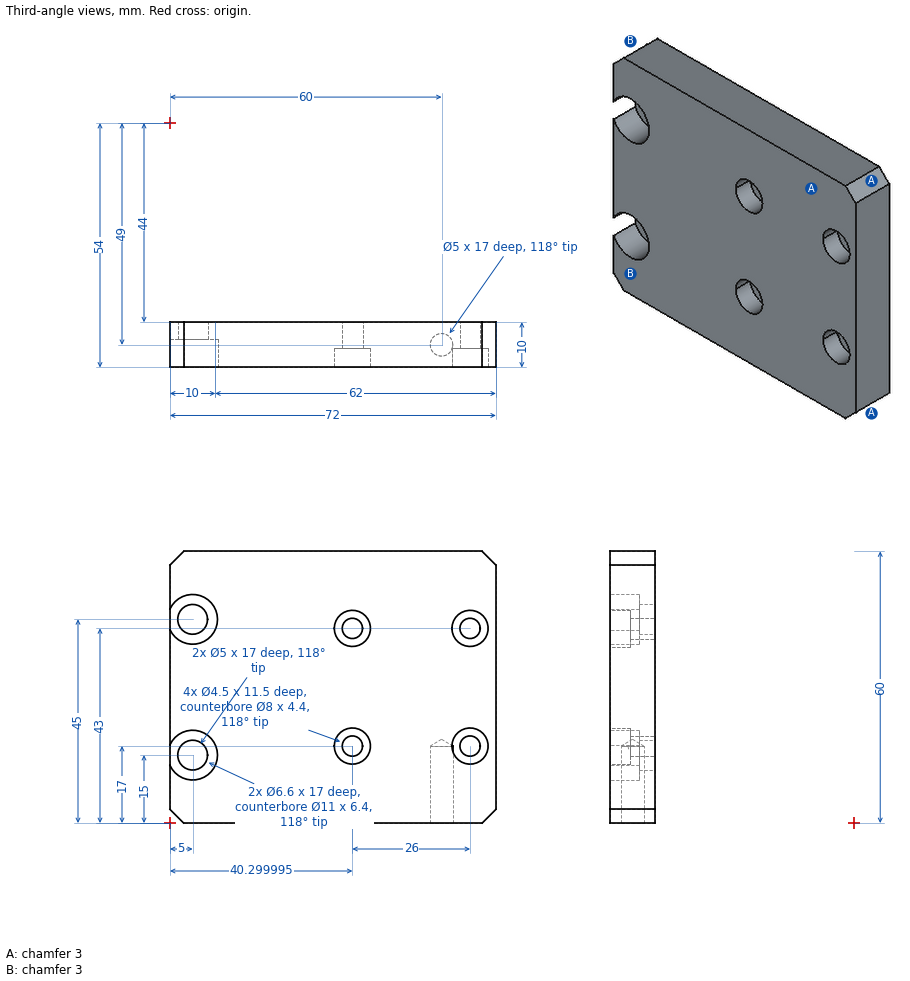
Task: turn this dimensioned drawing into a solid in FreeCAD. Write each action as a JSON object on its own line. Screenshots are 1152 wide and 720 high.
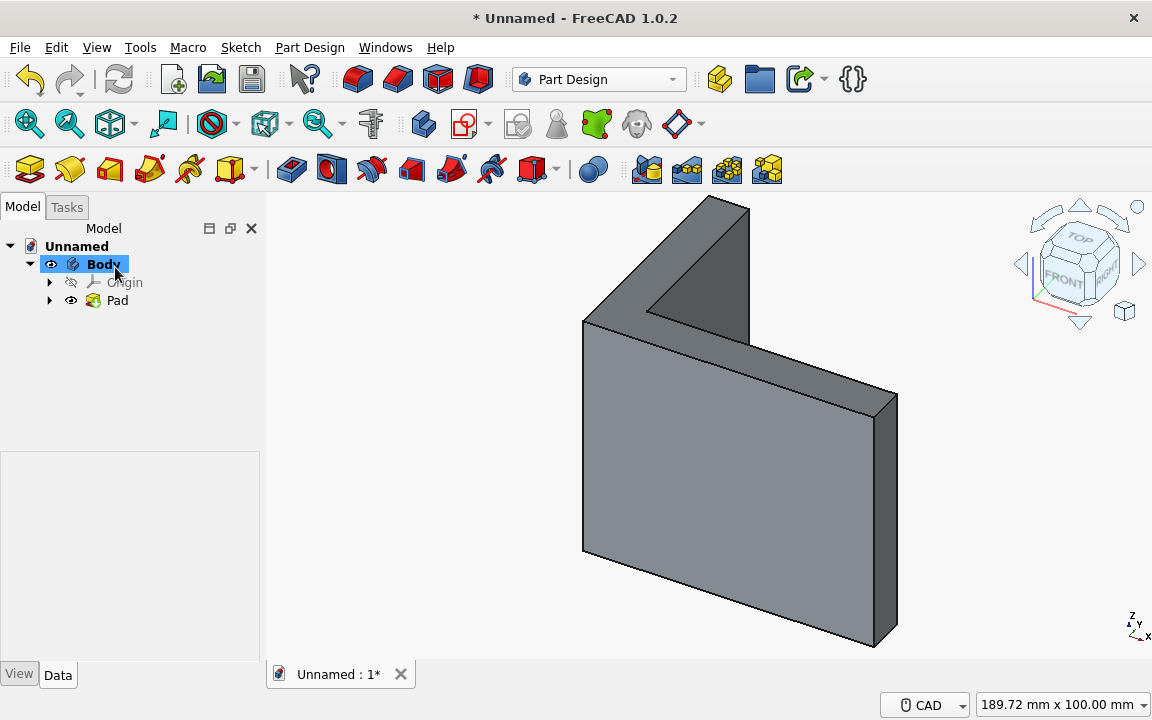
{"action": "key", "text": "5"}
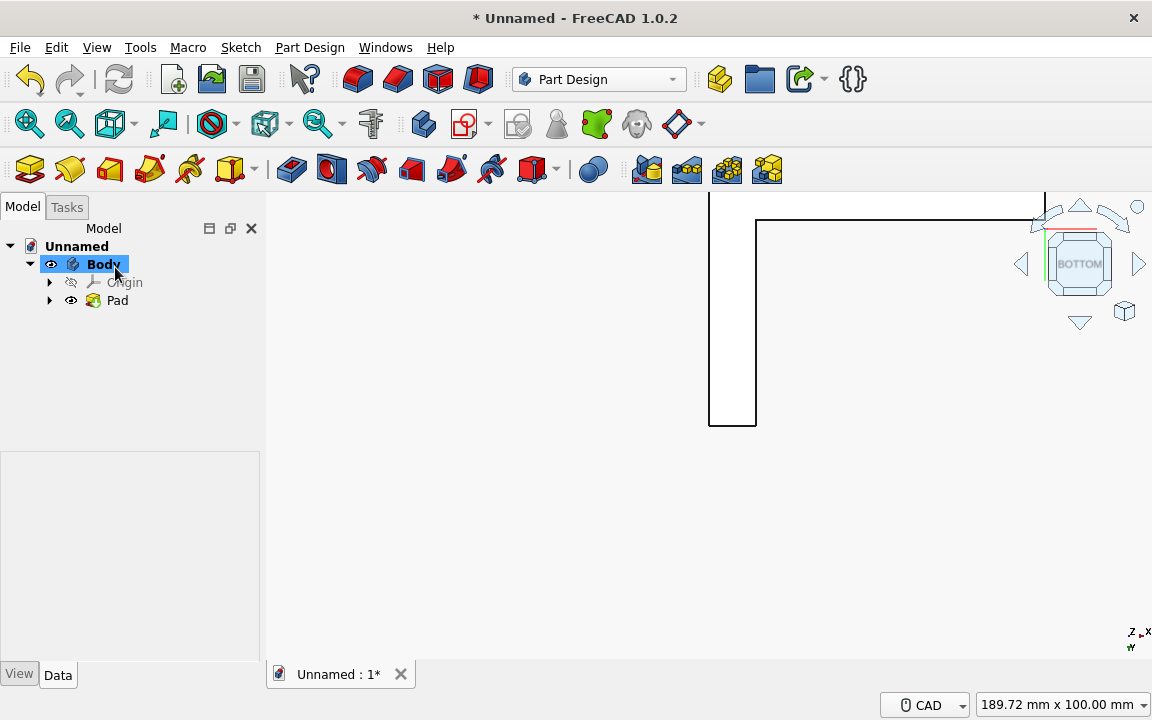
{"action": "left_click", "coordinate": [30, 124]}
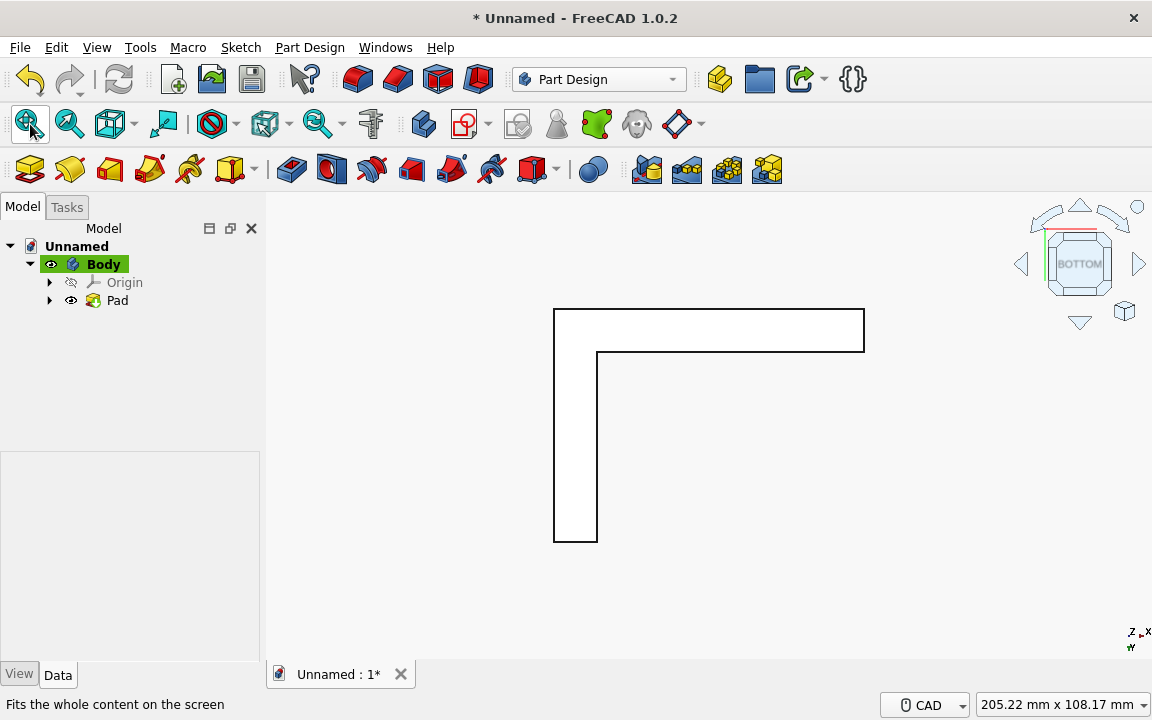
{"action": "left_click", "coordinate": [576, 491]}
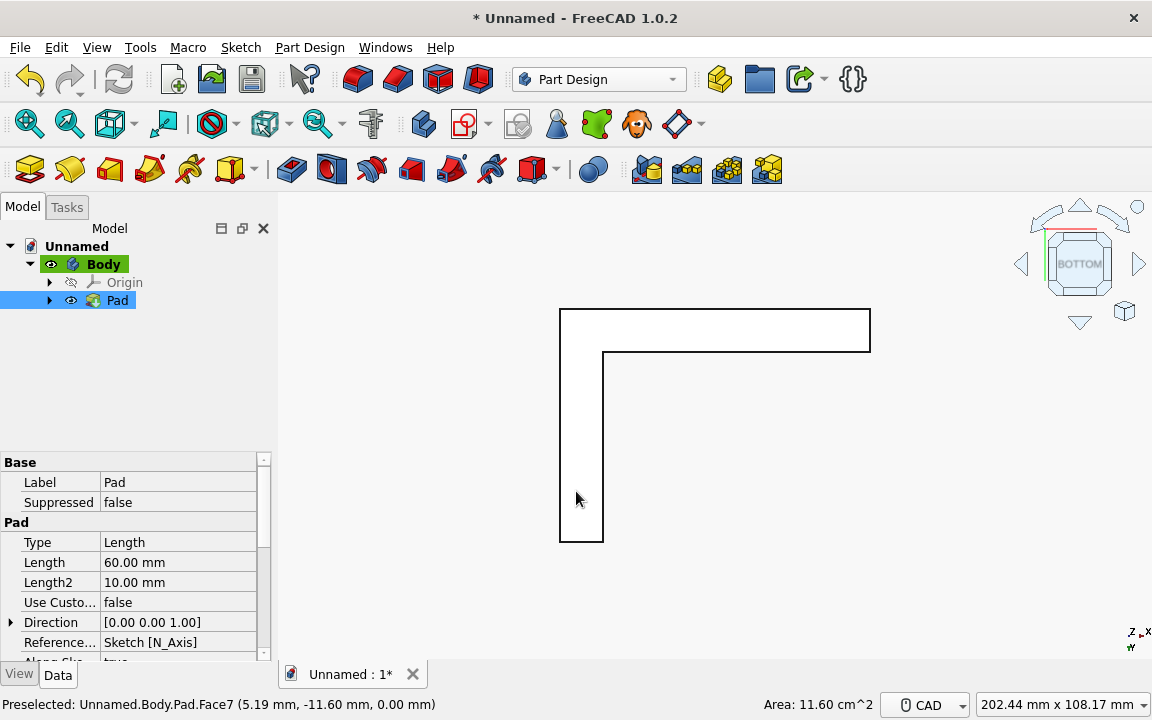
{"action": "left_click", "coordinate": [464, 124]}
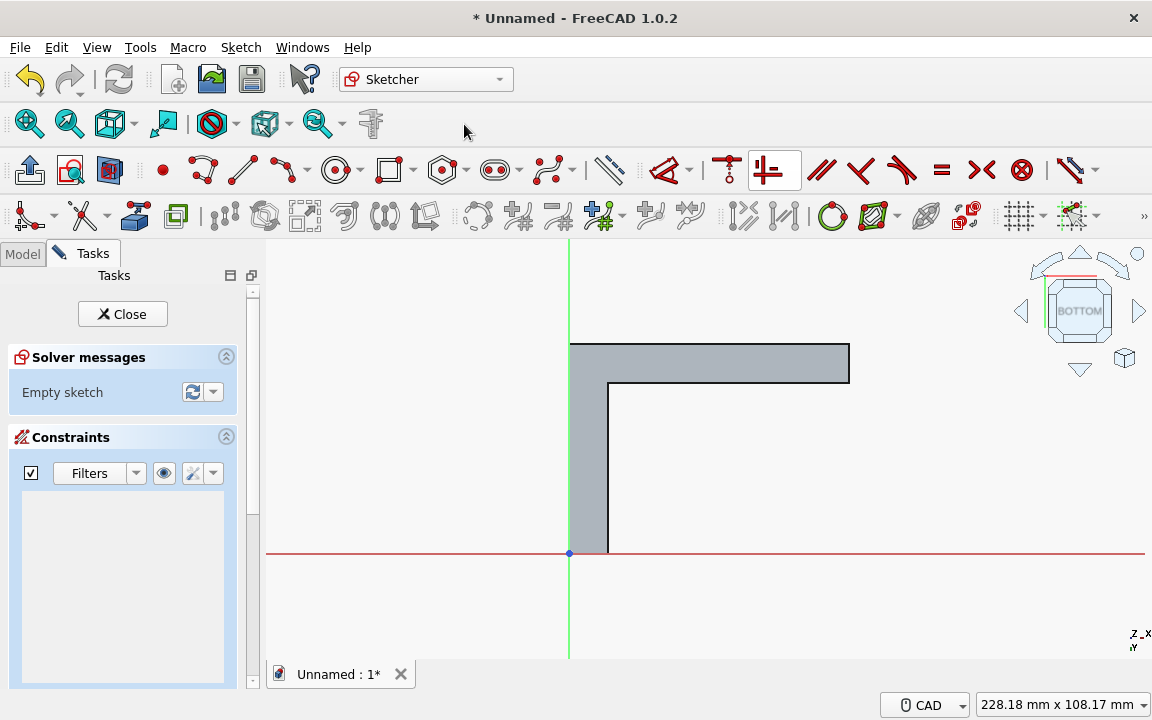
{"action": "scroll", "coordinate": [815, 357], "scroll_direction": "up", "scroll_amount": 13}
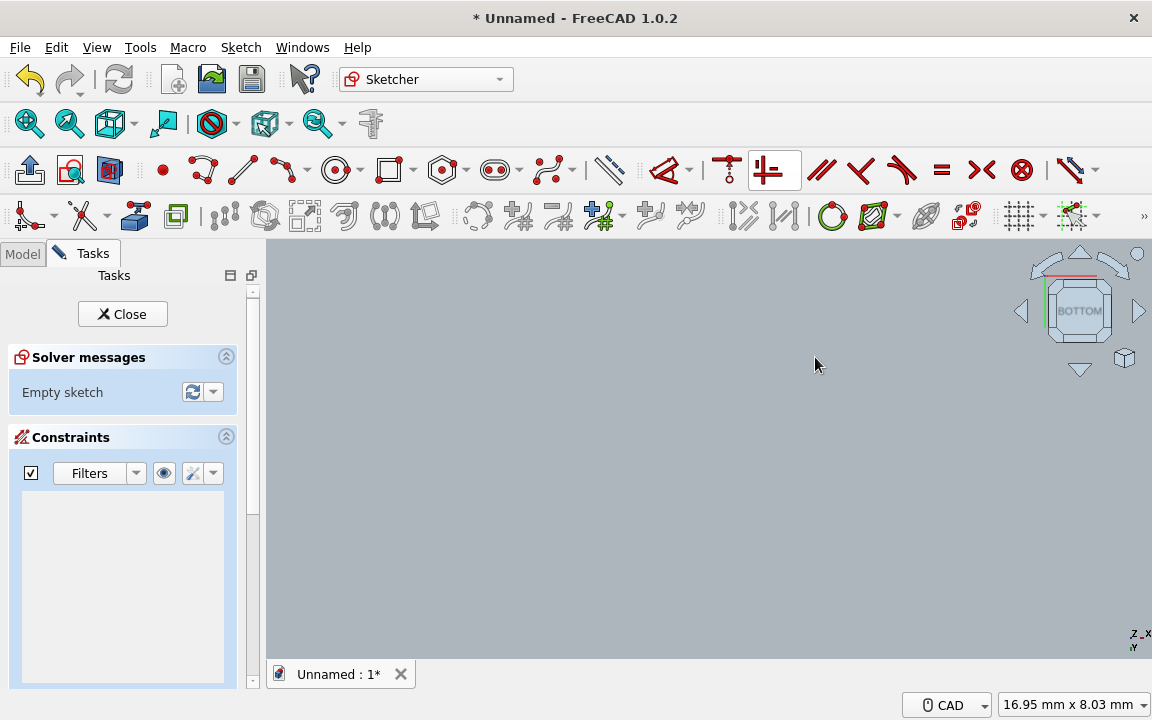
{"action": "left_click", "coordinate": [336, 170]}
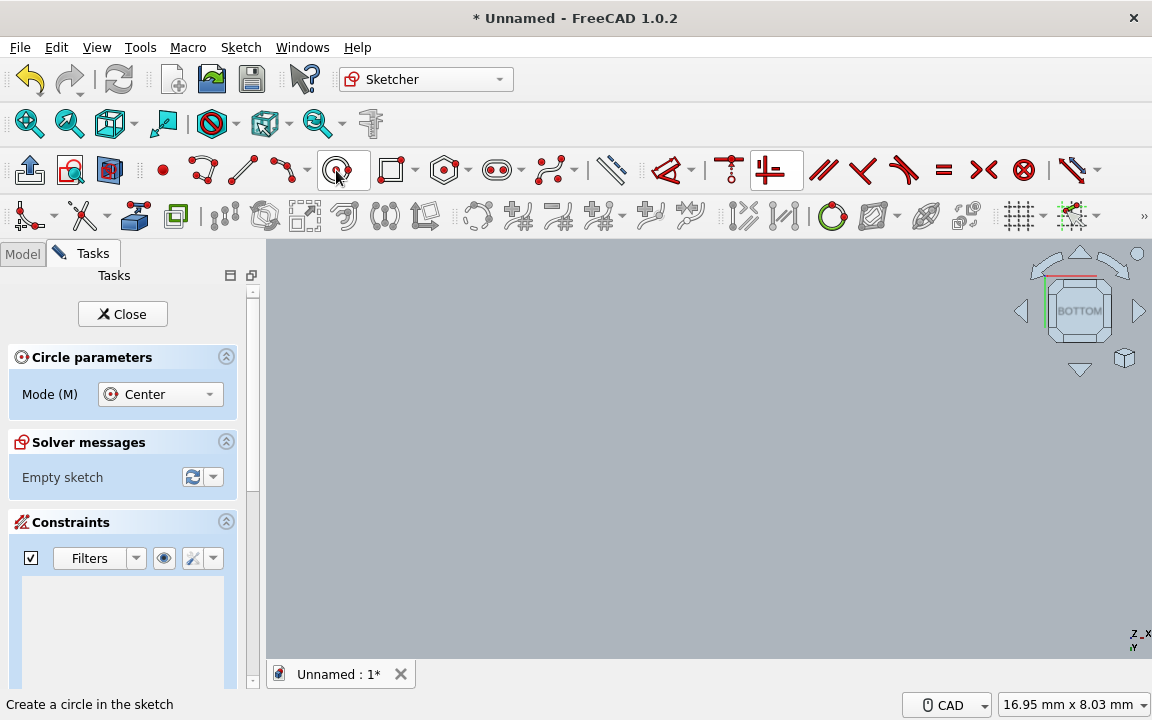
{"action": "left_click", "coordinate": [635, 442]}
{"action": "left_click", "coordinate": [727, 350]}
{"action": "key", "text": "Escape"}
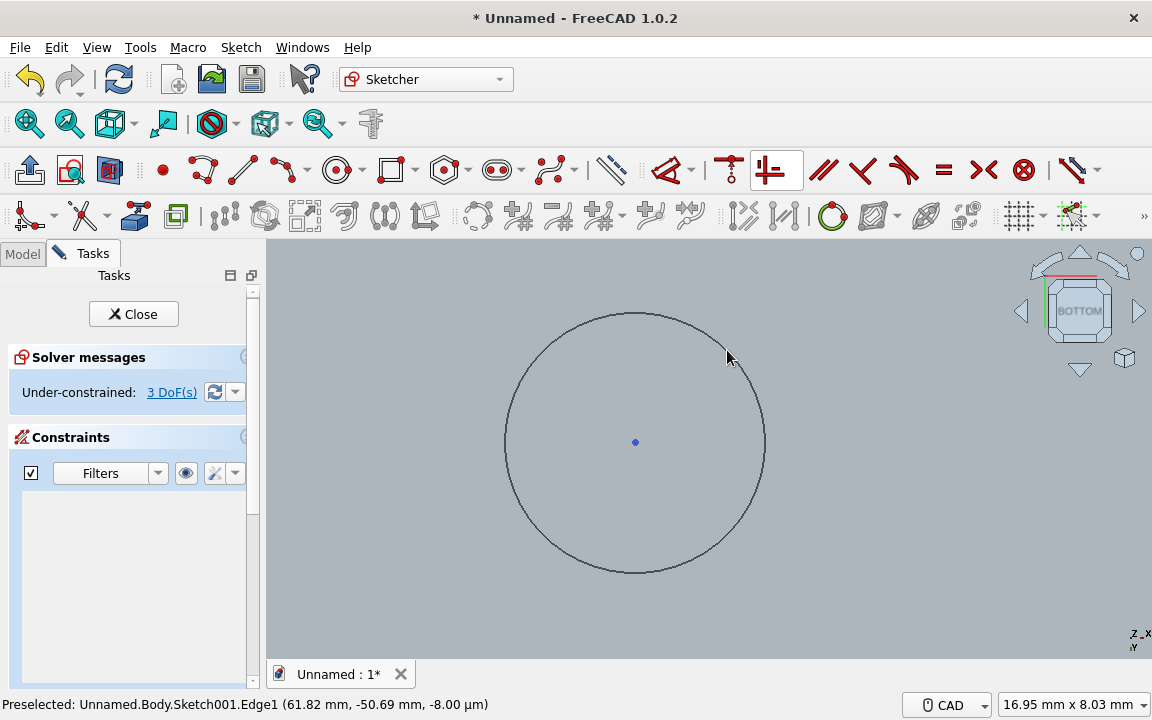
{"action": "left_click", "coordinate": [666, 170]}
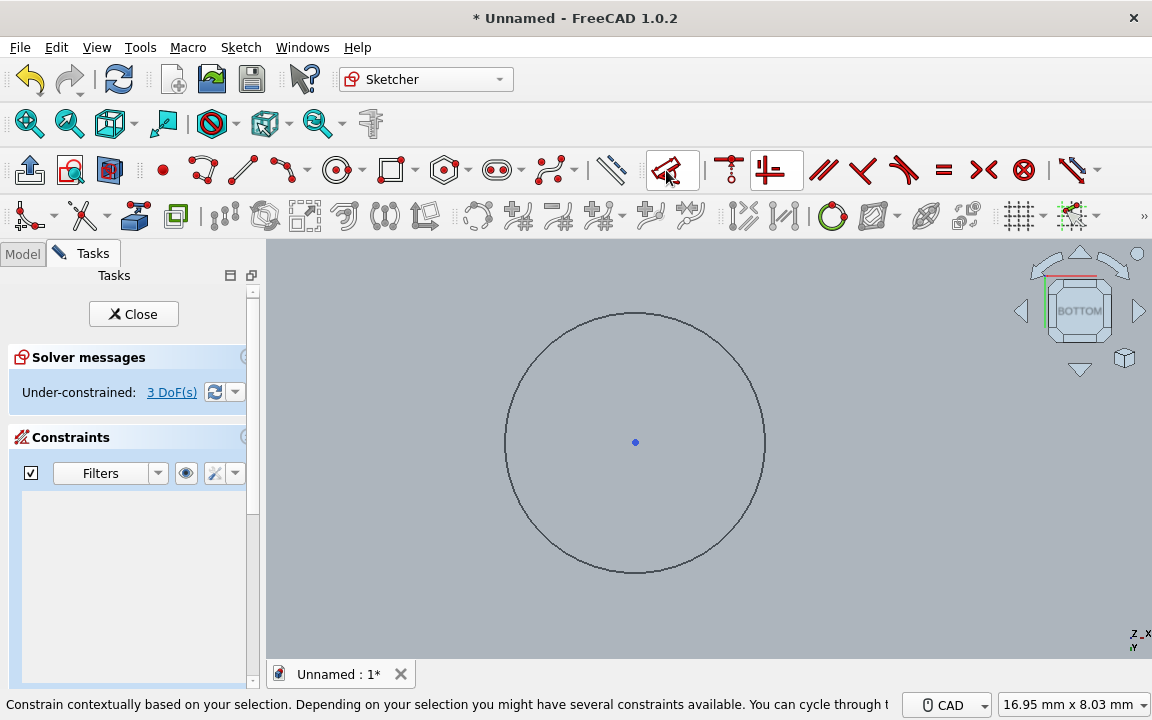
{"action": "left_click", "coordinate": [727, 351]}
{"action": "left_click", "coordinate": [750, 328]}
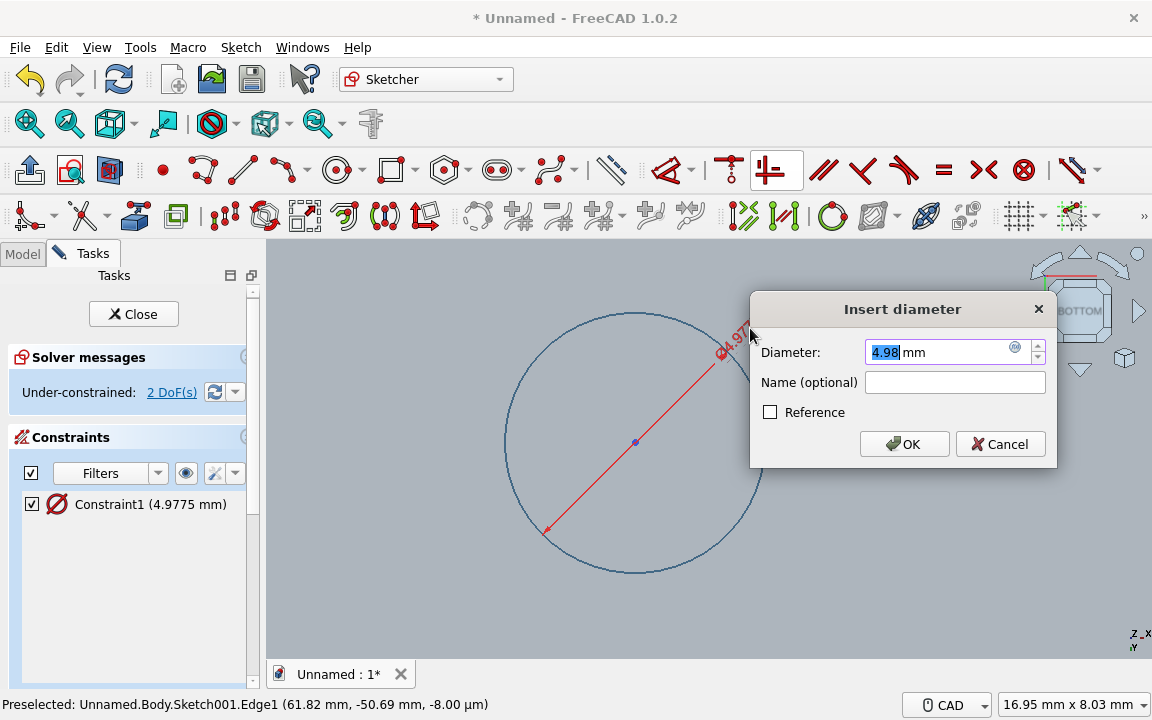
{"action": "type", "text": "5"}
{"action": "key", "text": "Return"}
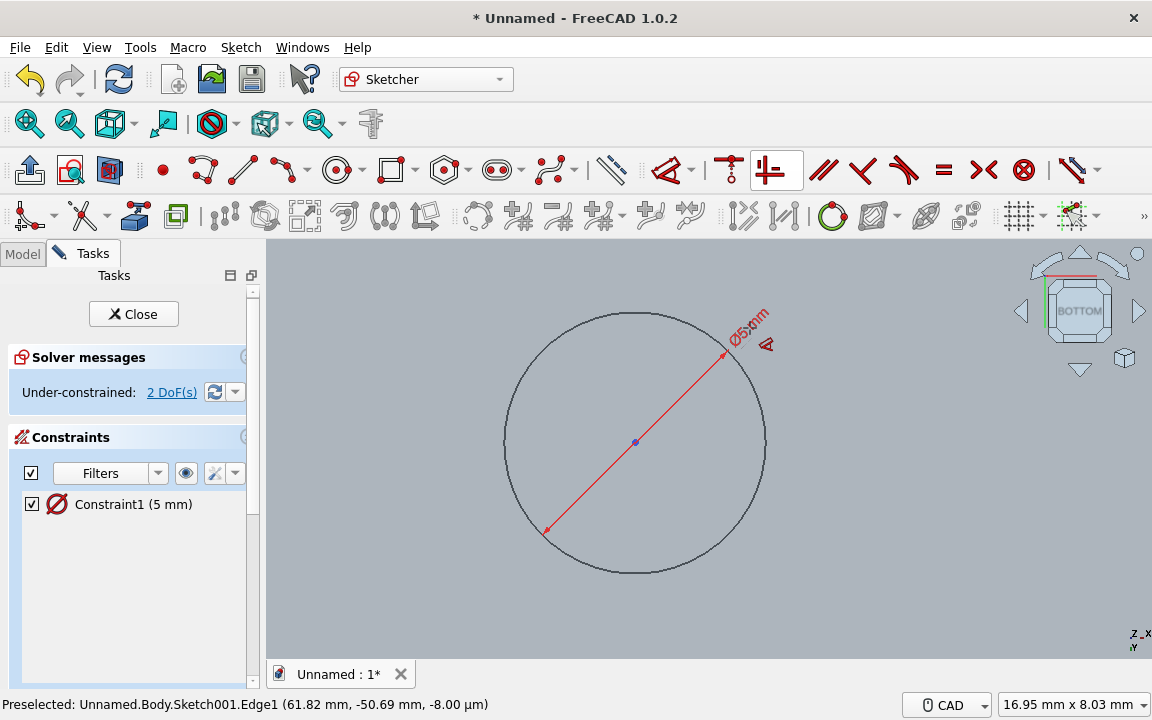
{"action": "left_click", "coordinate": [635, 443]}
{"action": "left_click", "coordinate": [464, 409]}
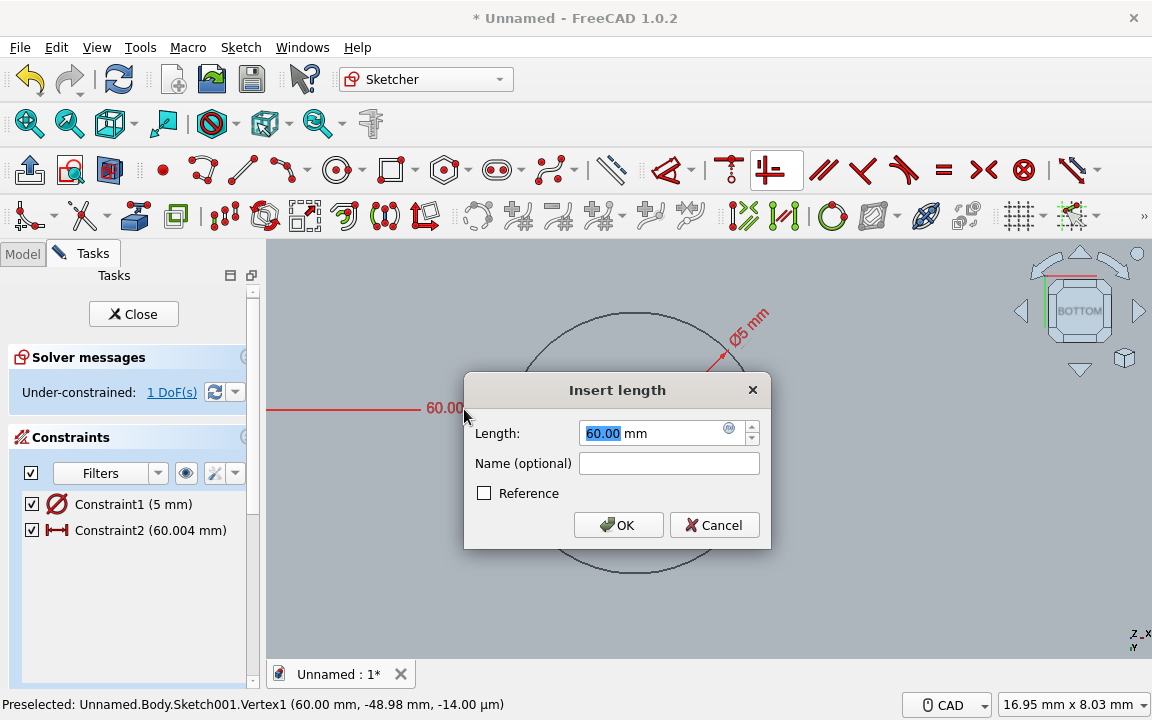
{"action": "type", "text": "60"}
{"action": "key", "text": "Return"}